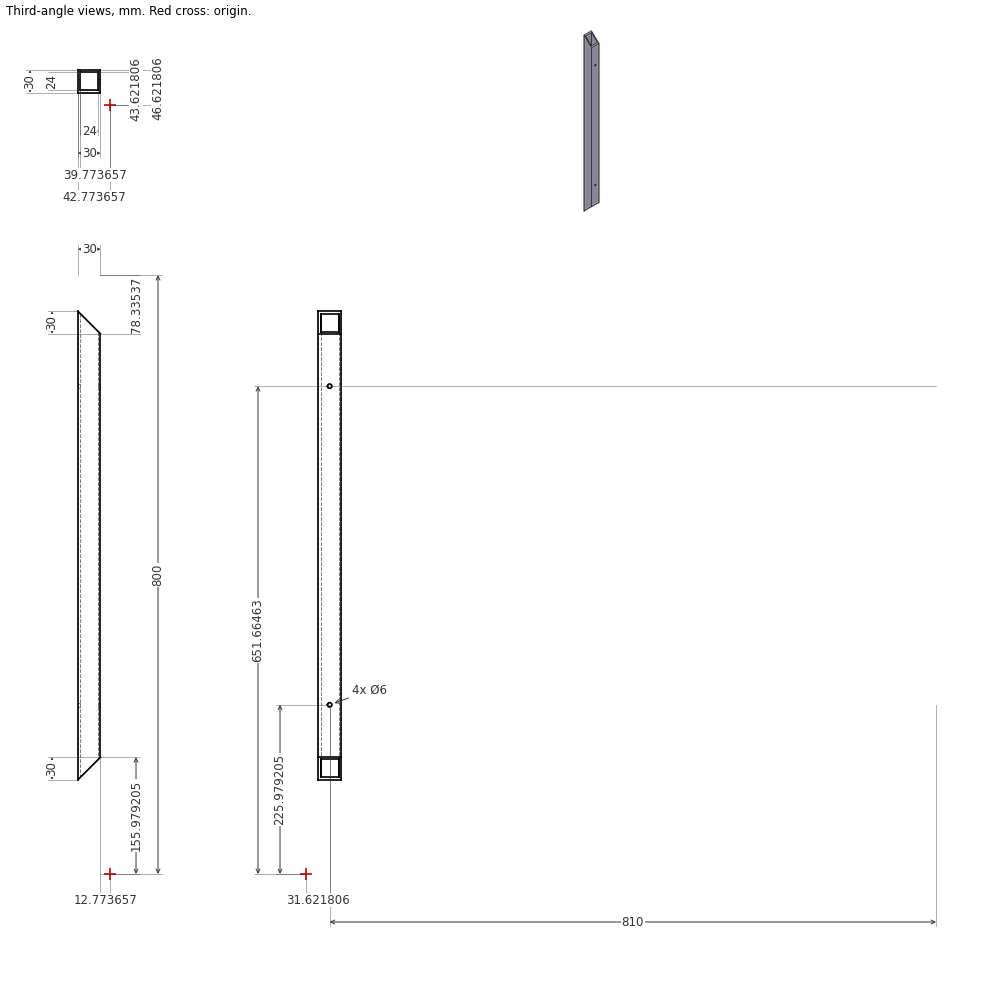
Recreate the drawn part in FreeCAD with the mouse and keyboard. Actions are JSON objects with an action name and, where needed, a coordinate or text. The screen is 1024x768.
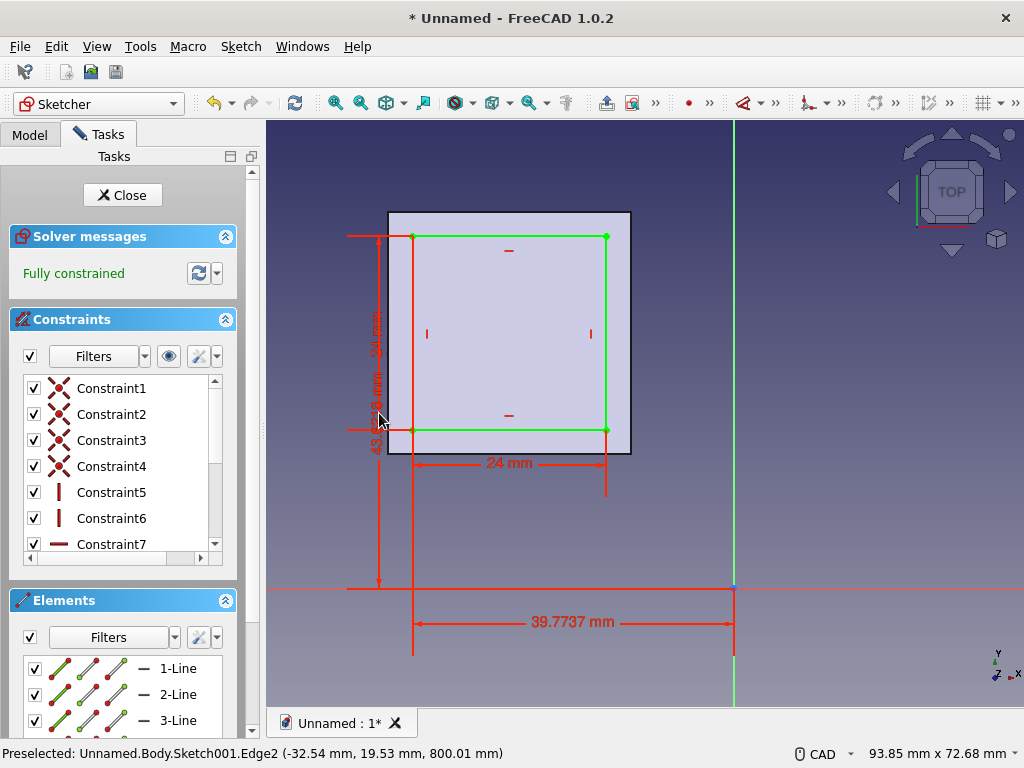
{"action": "left_click", "coordinate": [123, 195]}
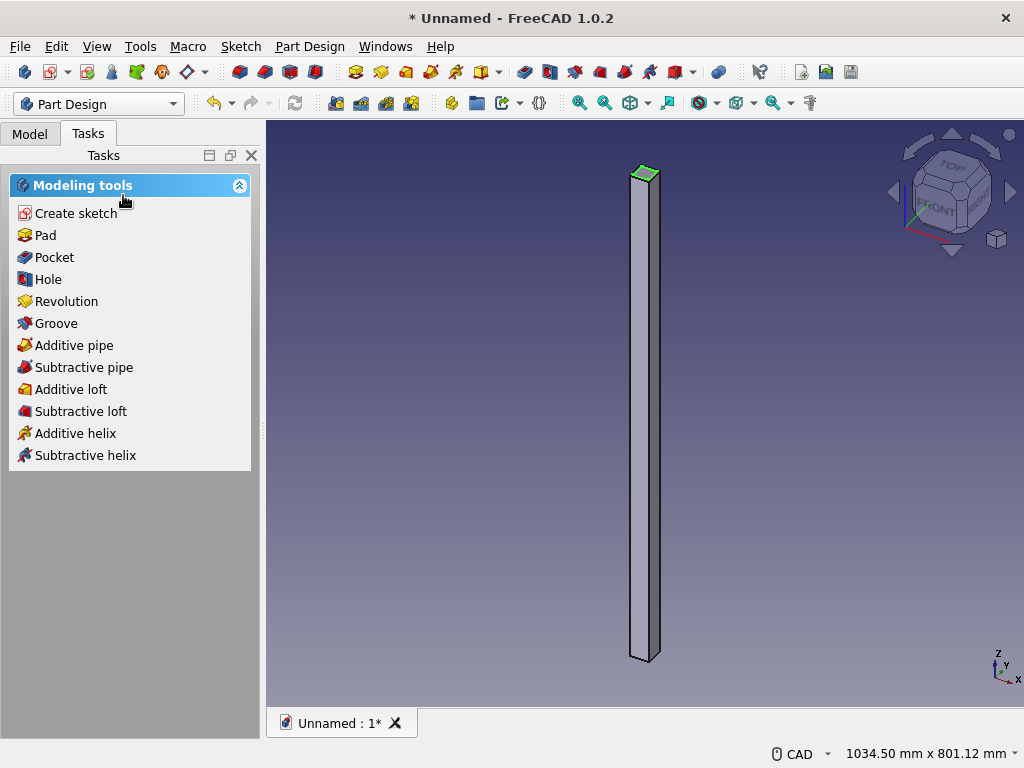
{"action": "left_click", "coordinate": [525, 72]}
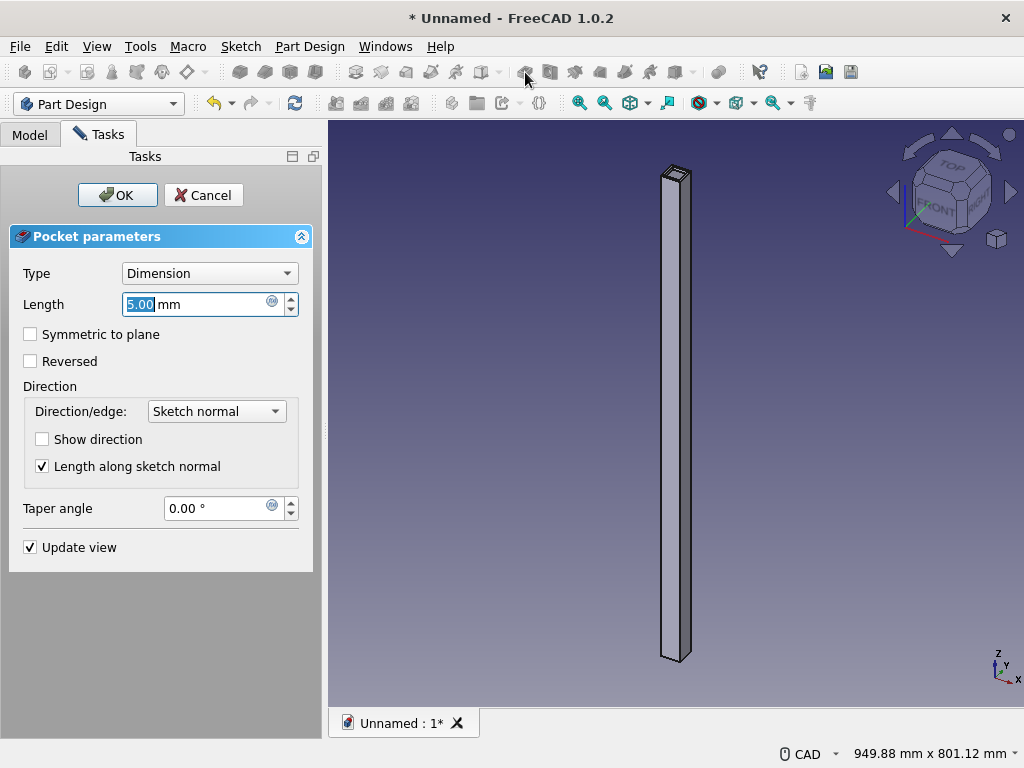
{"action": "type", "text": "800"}
{"action": "key", "text": "Tab"}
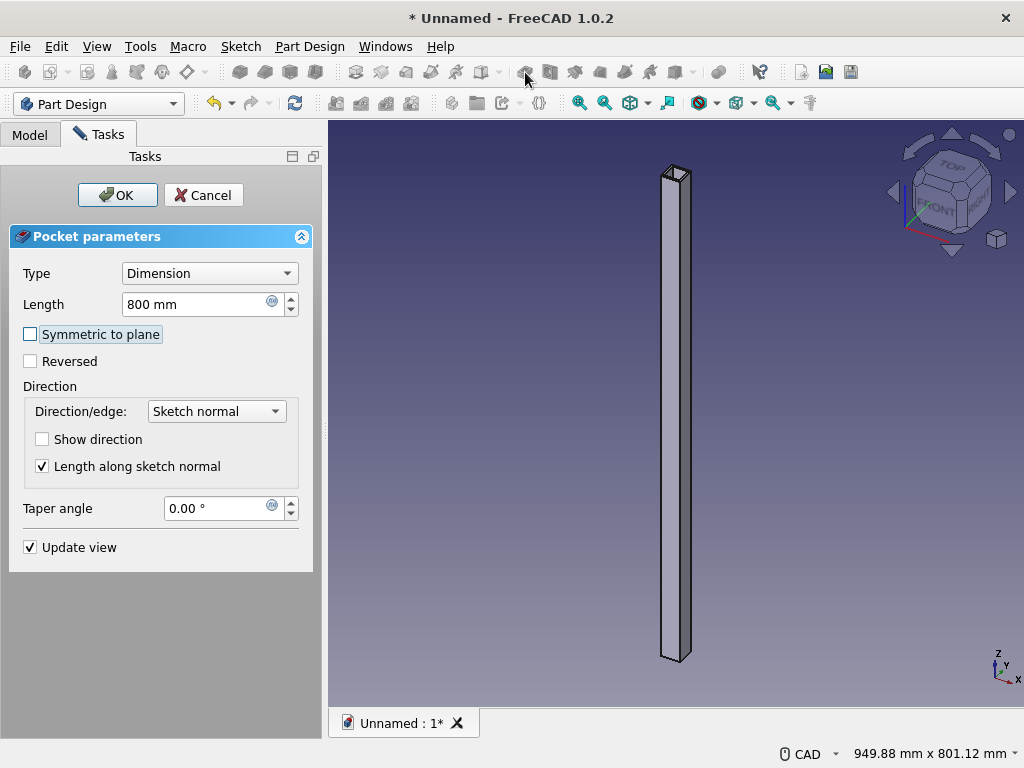
{"action": "left_click", "coordinate": [118, 195]}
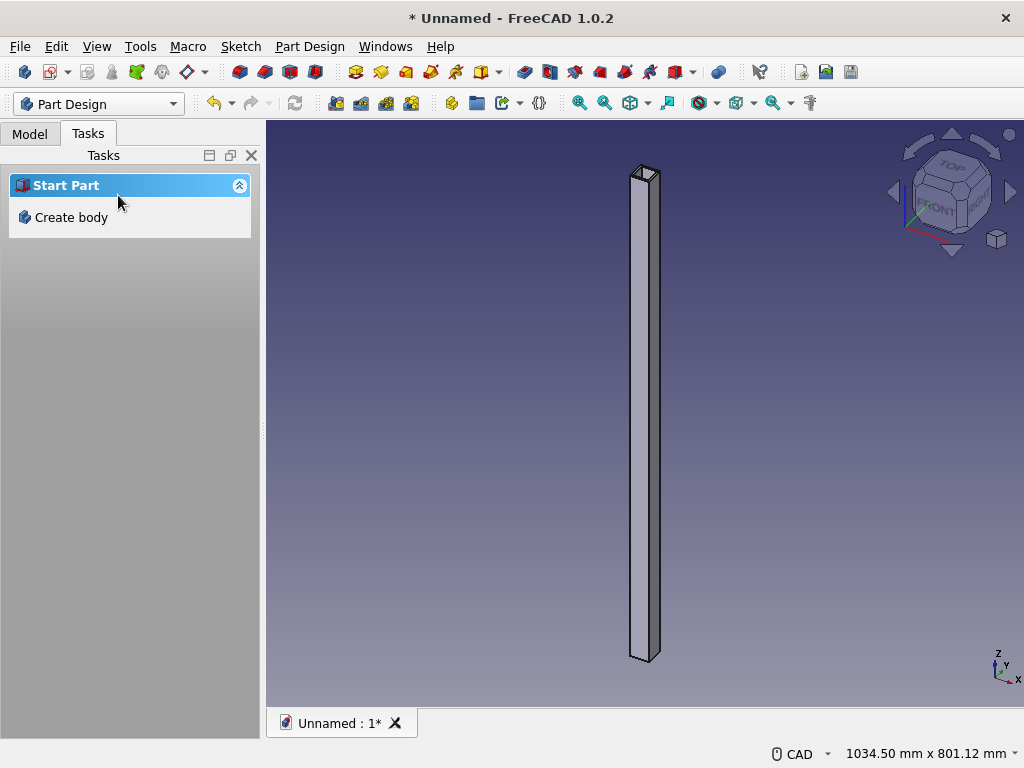
{"action": "left_click", "coordinate": [640, 212]}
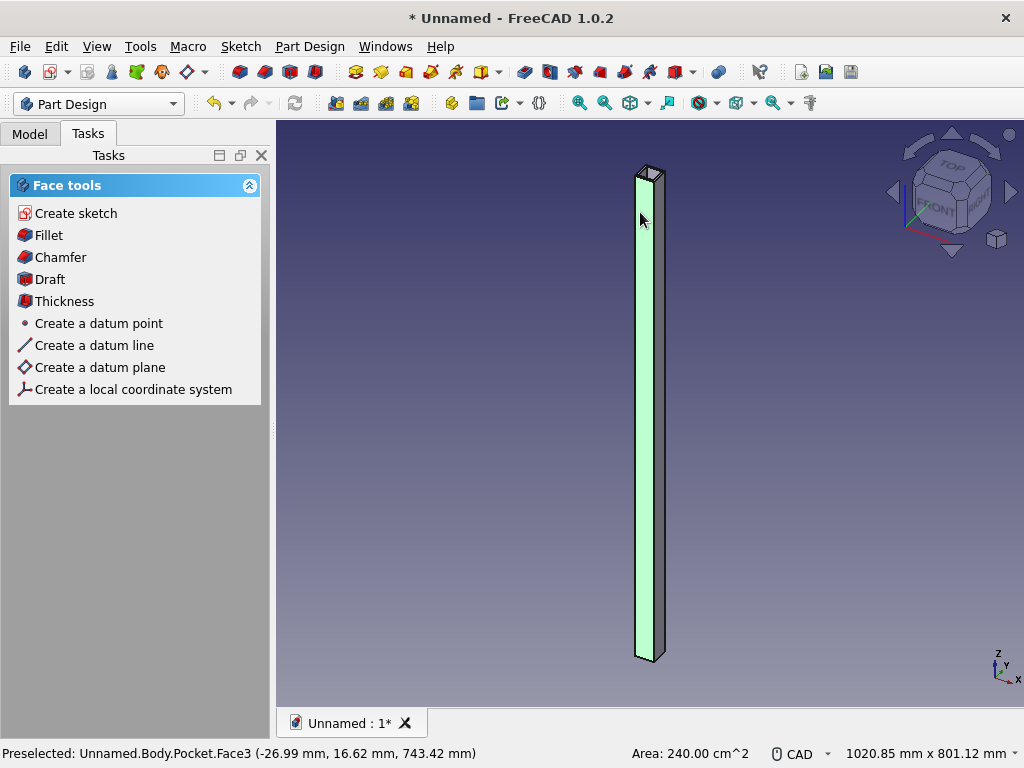
{"action": "left_click", "coordinate": [50, 72]}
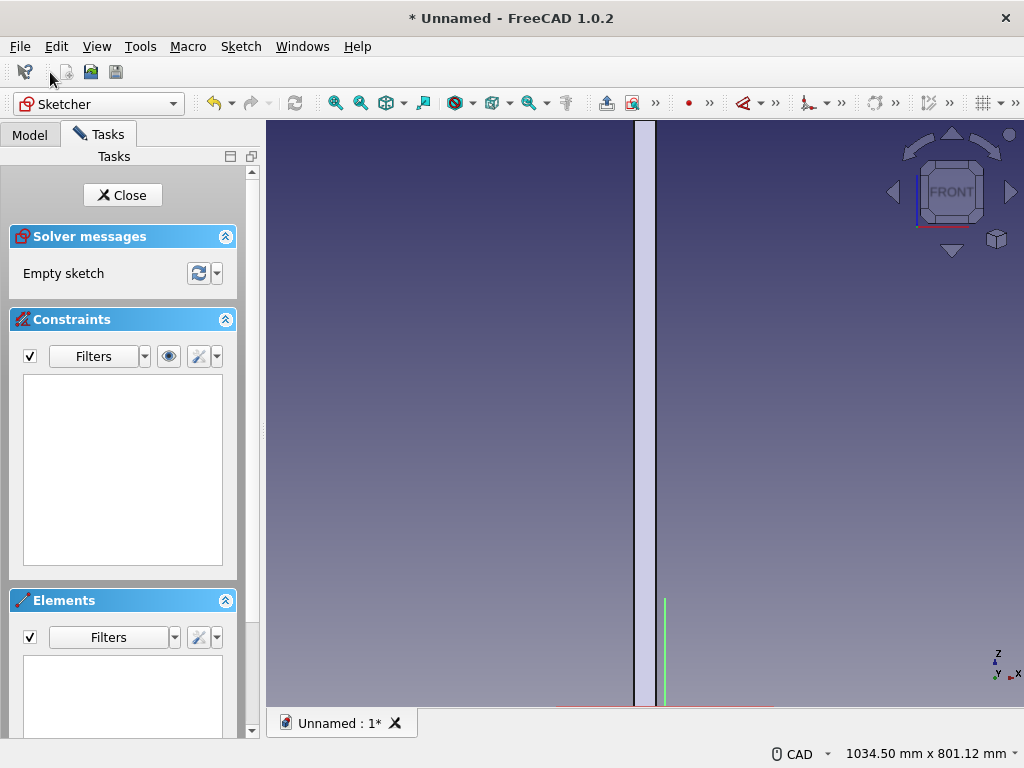
{"action": "scroll", "coordinate": [428, 413], "scroll_direction": "down", "scroll_amount": 2}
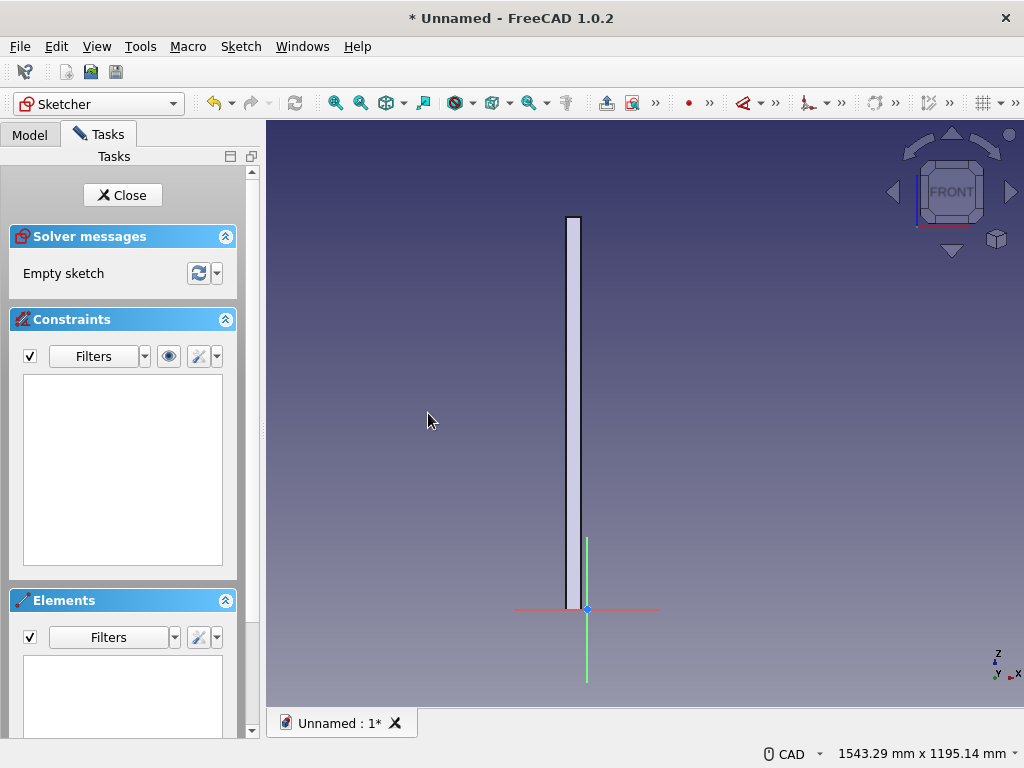
{"action": "key", "text": "g m"}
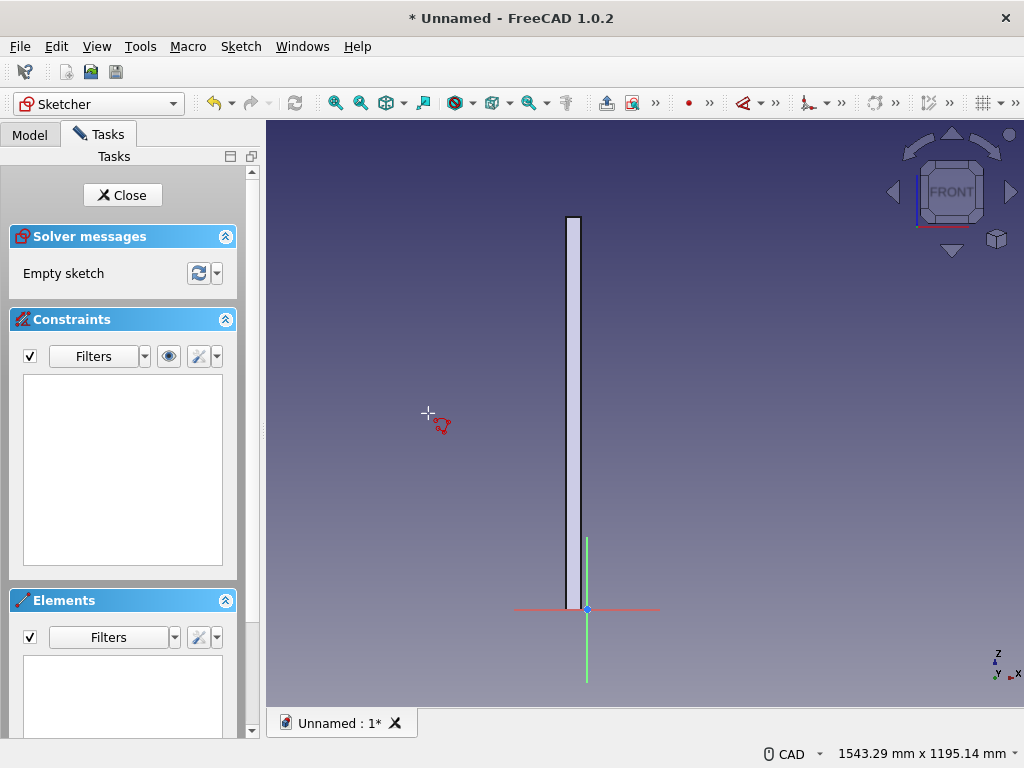
{"action": "scroll", "coordinate": [581, 256], "scroll_direction": "up", "scroll_amount": 5}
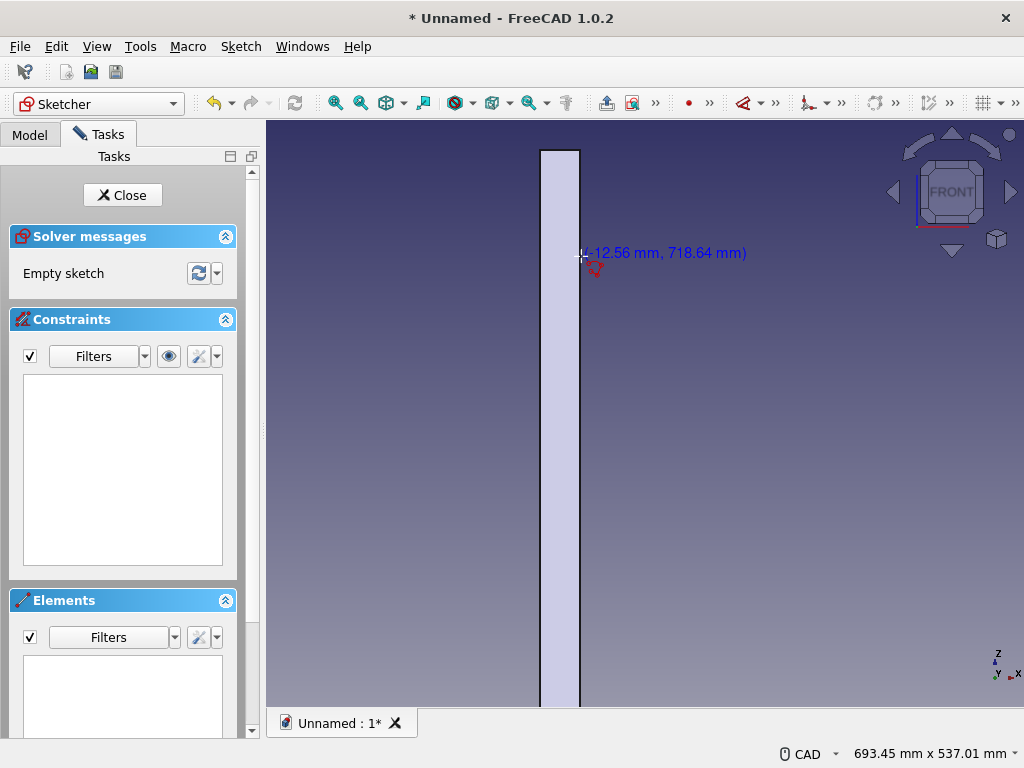
{"action": "left_click", "coordinate": [580, 254]}
{"action": "left_click", "coordinate": [580, 150]}
{"action": "left_click", "coordinate": [540, 150]}
{"action": "left_click", "coordinate": [540, 214]}
{"action": "left_click", "coordinate": [580, 255]}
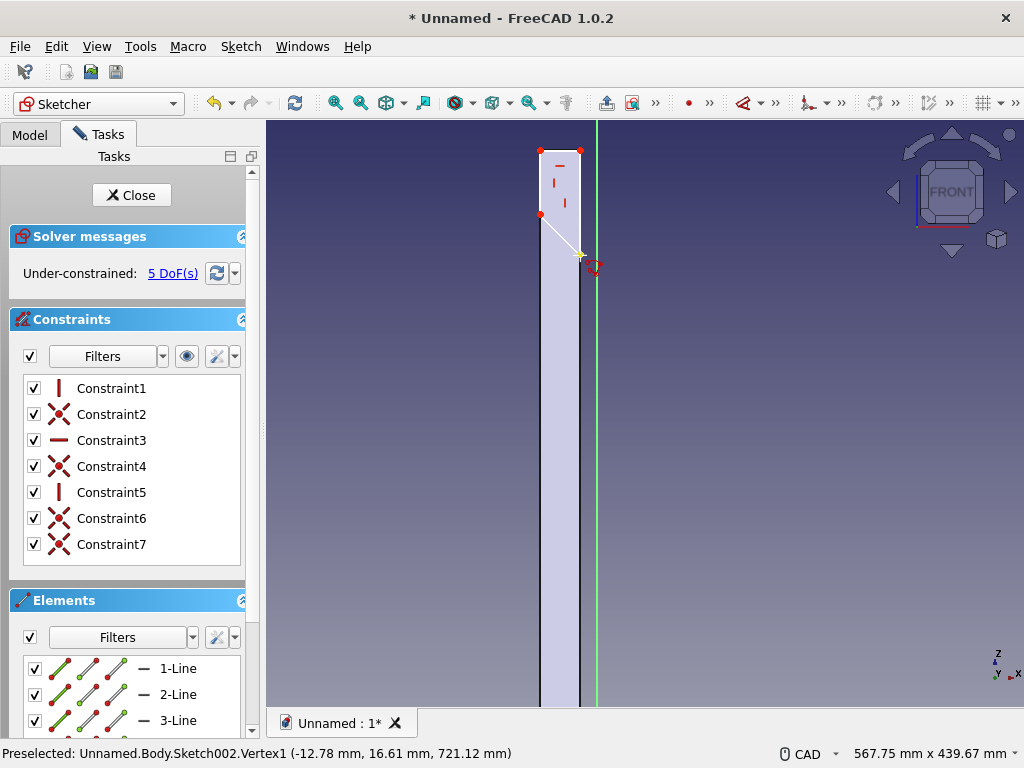
{"action": "scroll", "coordinate": [581, 256], "scroll_direction": "down", "scroll_amount": 5}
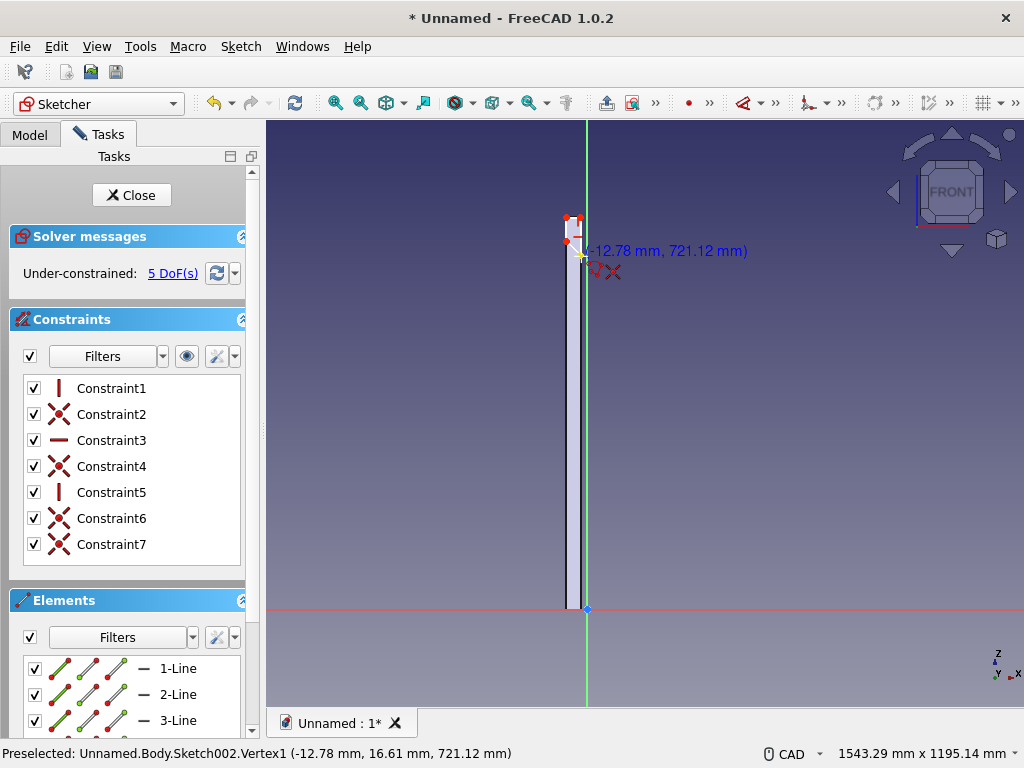
{"action": "scroll", "coordinate": [581, 610], "scroll_direction": "up", "scroll_amount": 5}